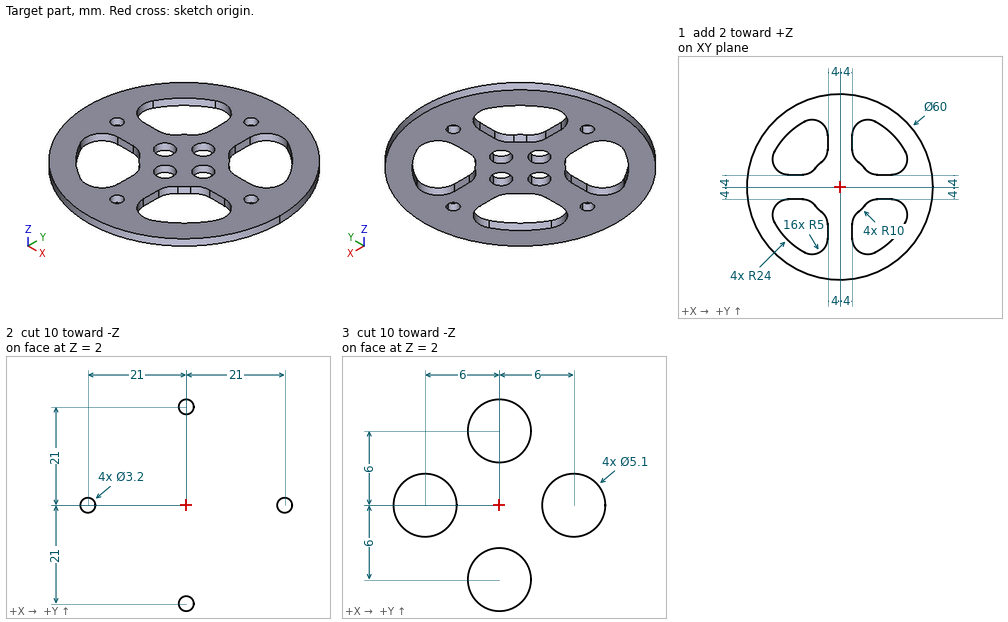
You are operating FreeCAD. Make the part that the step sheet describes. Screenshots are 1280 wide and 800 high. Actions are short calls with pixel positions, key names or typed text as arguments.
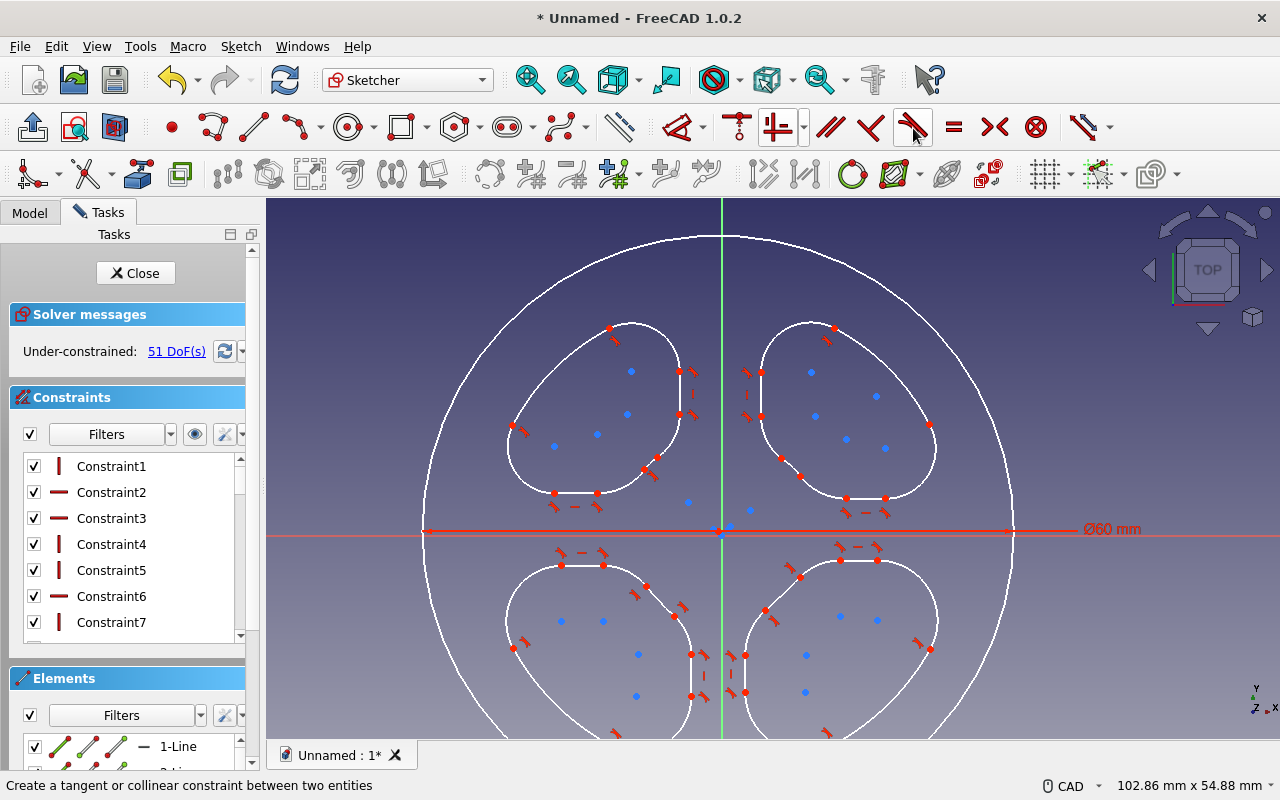
click(908, 390)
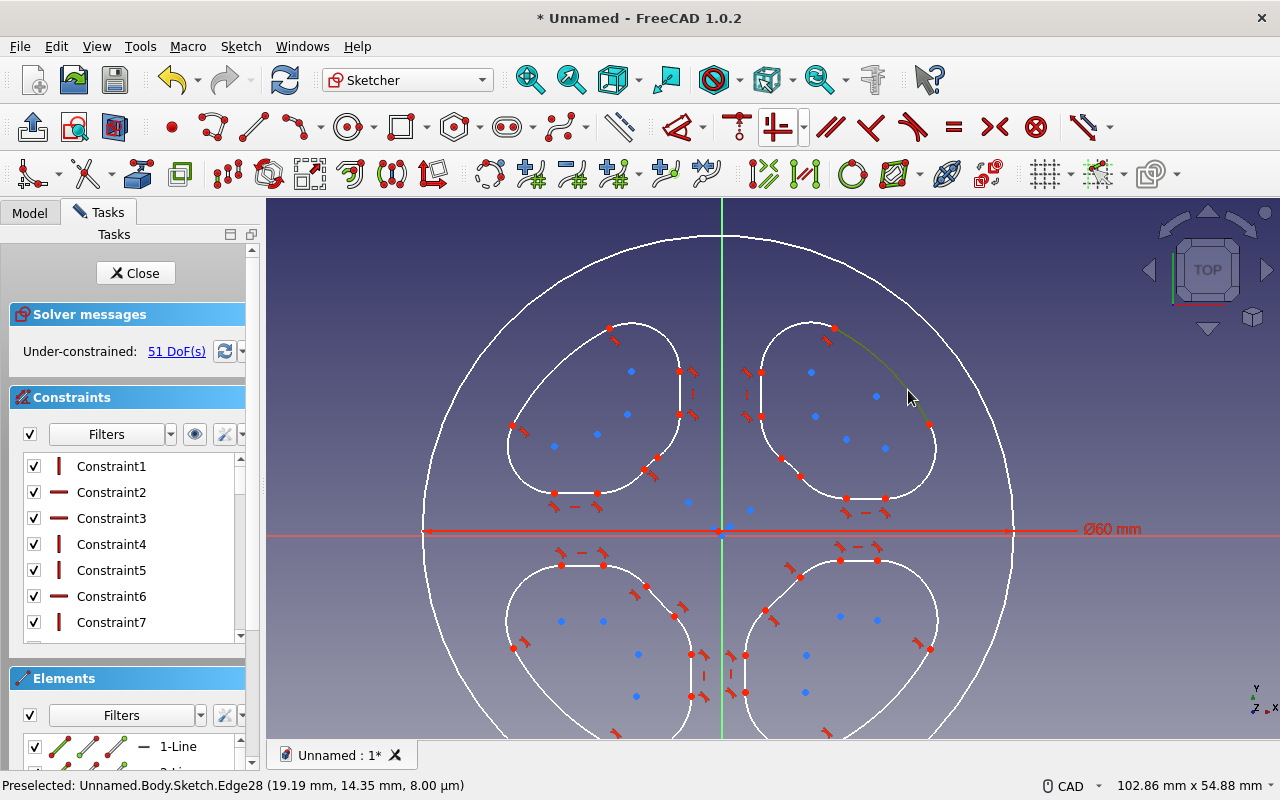
click(915, 489)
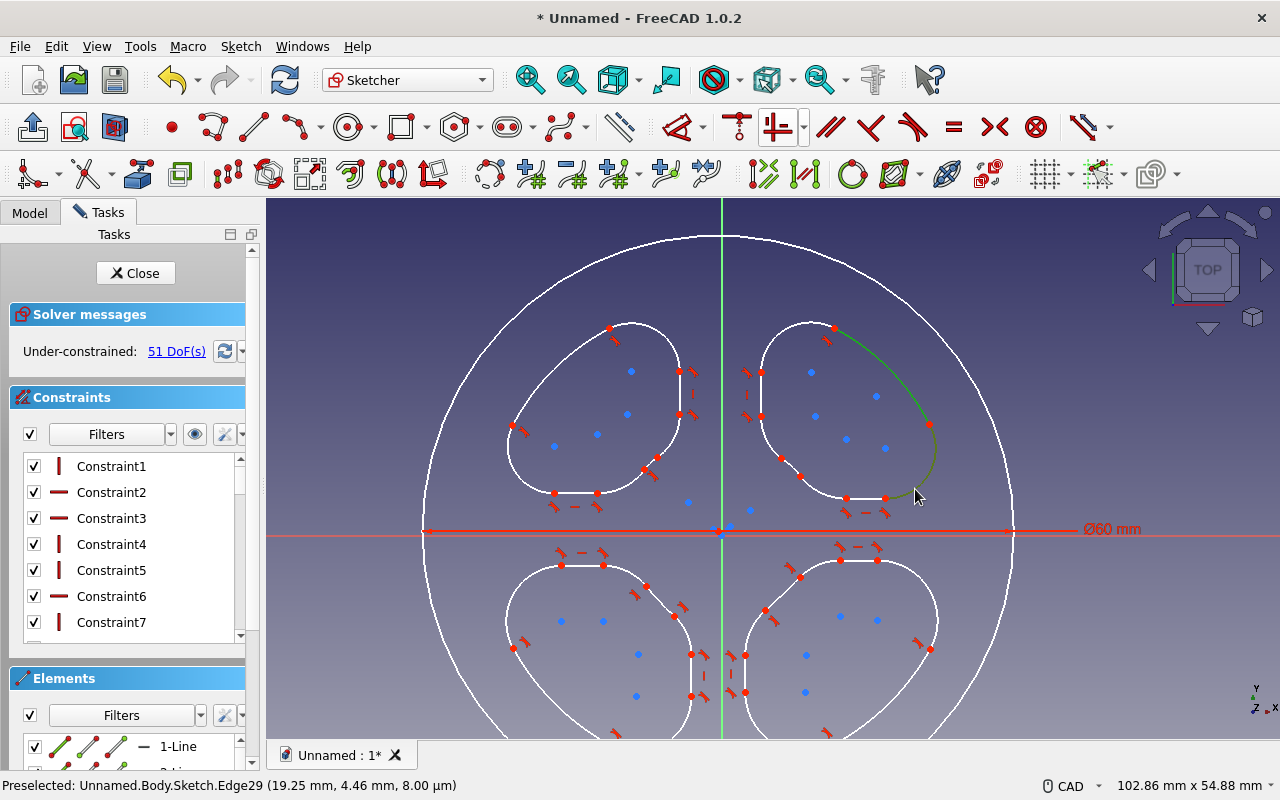
click(913, 128)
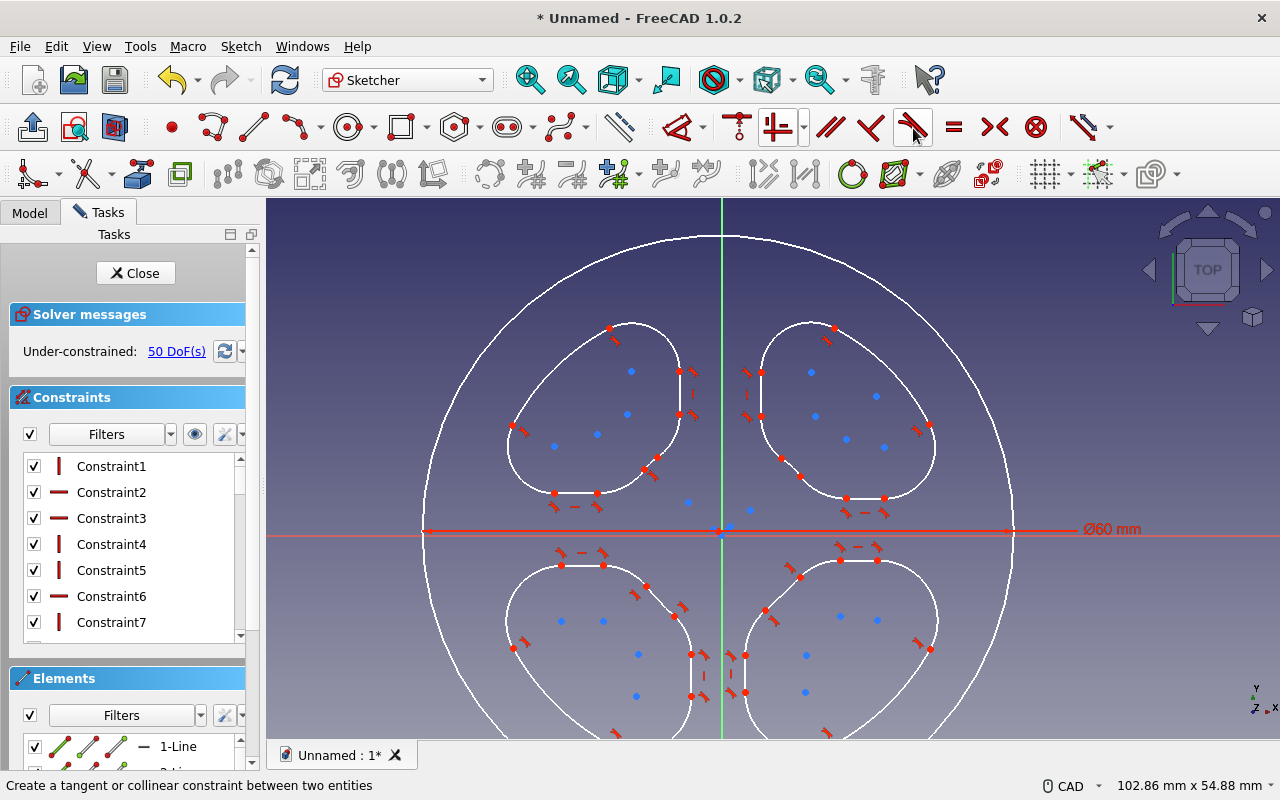
click(812, 488)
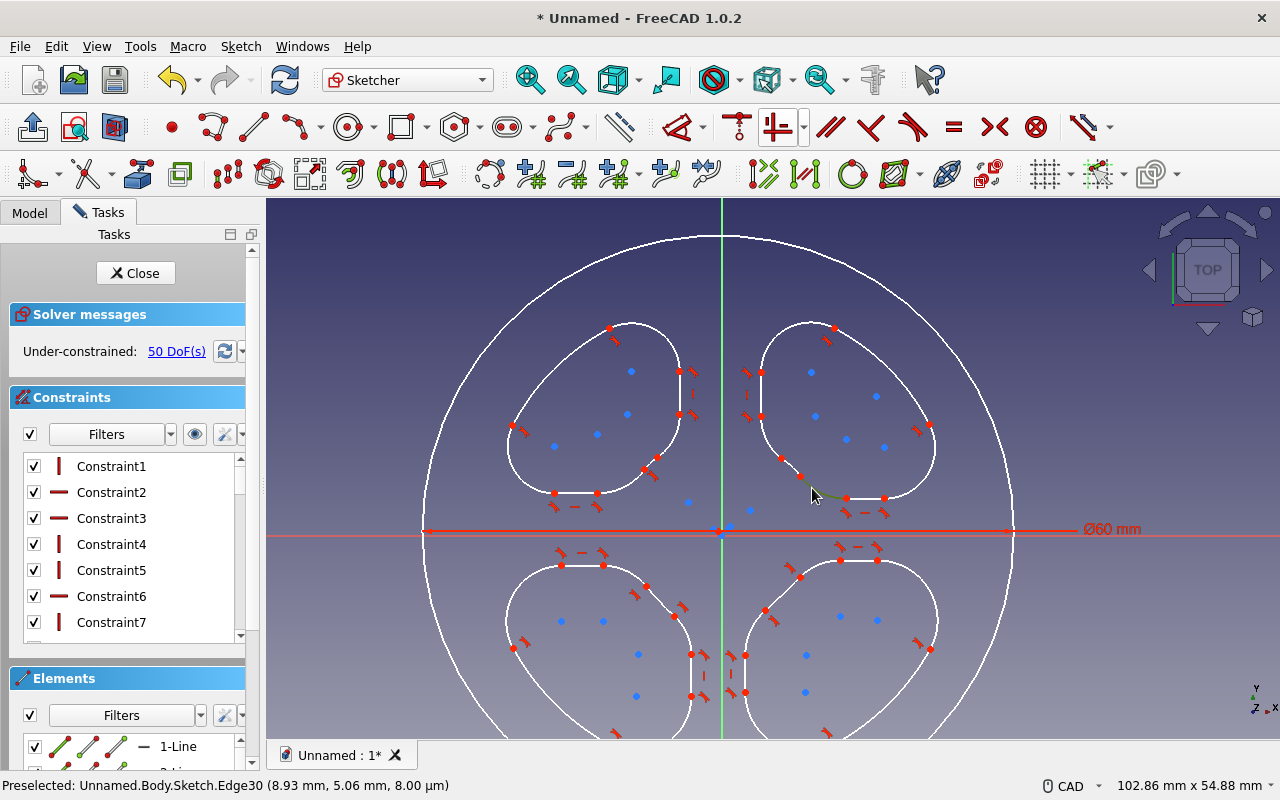
click(792, 467)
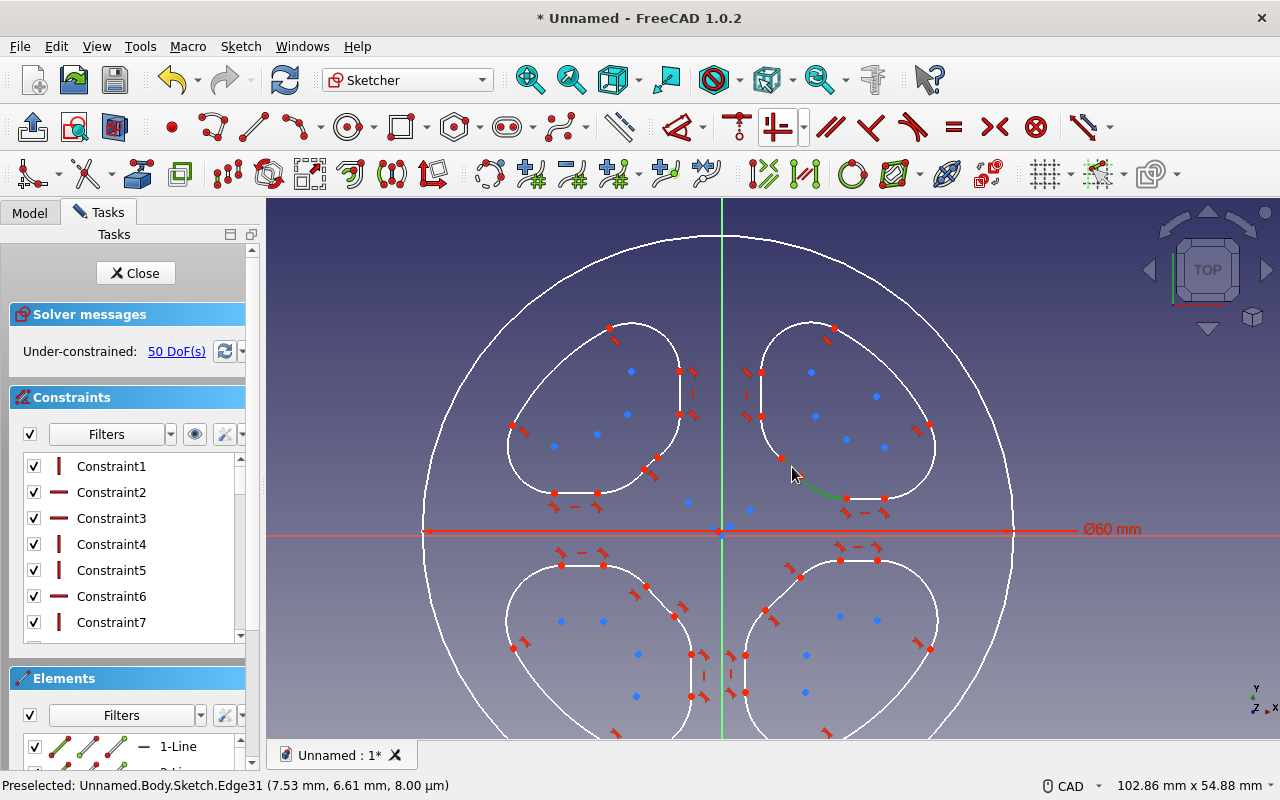
click(913, 128)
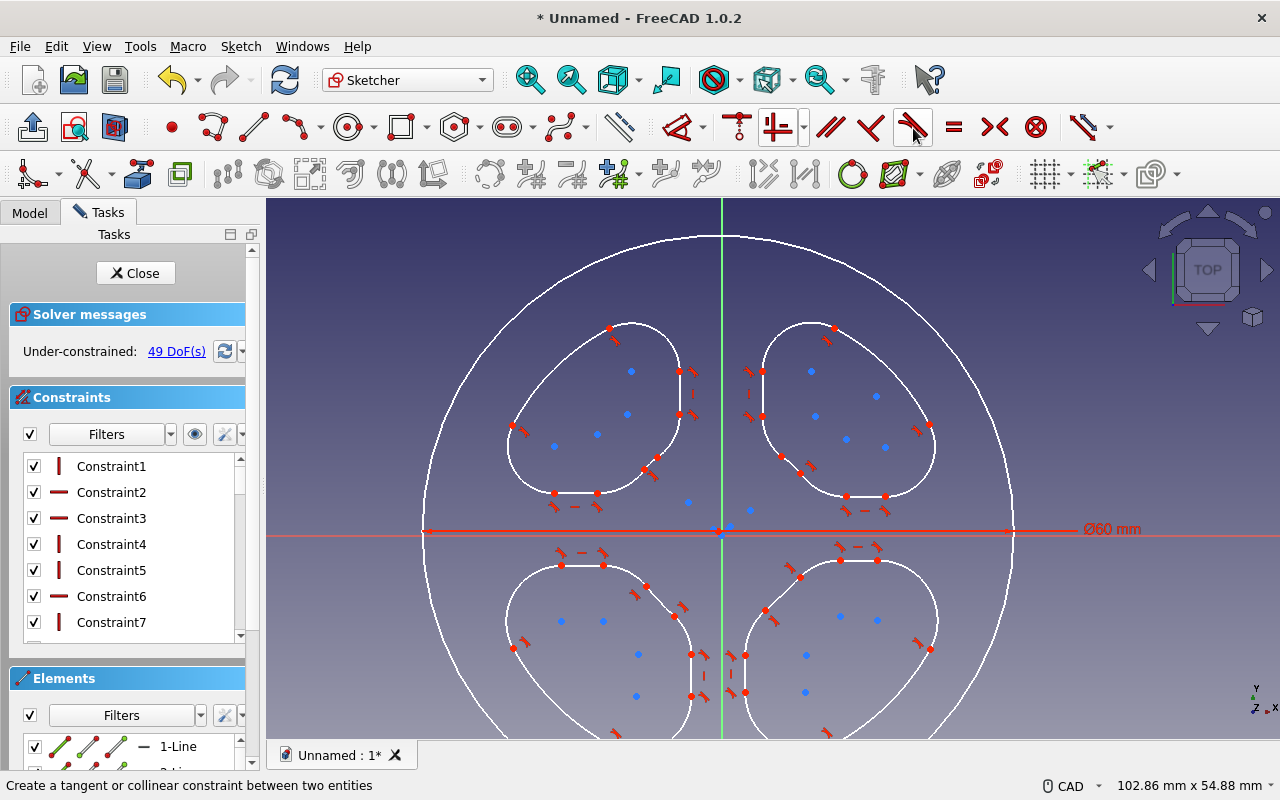
click(792, 464)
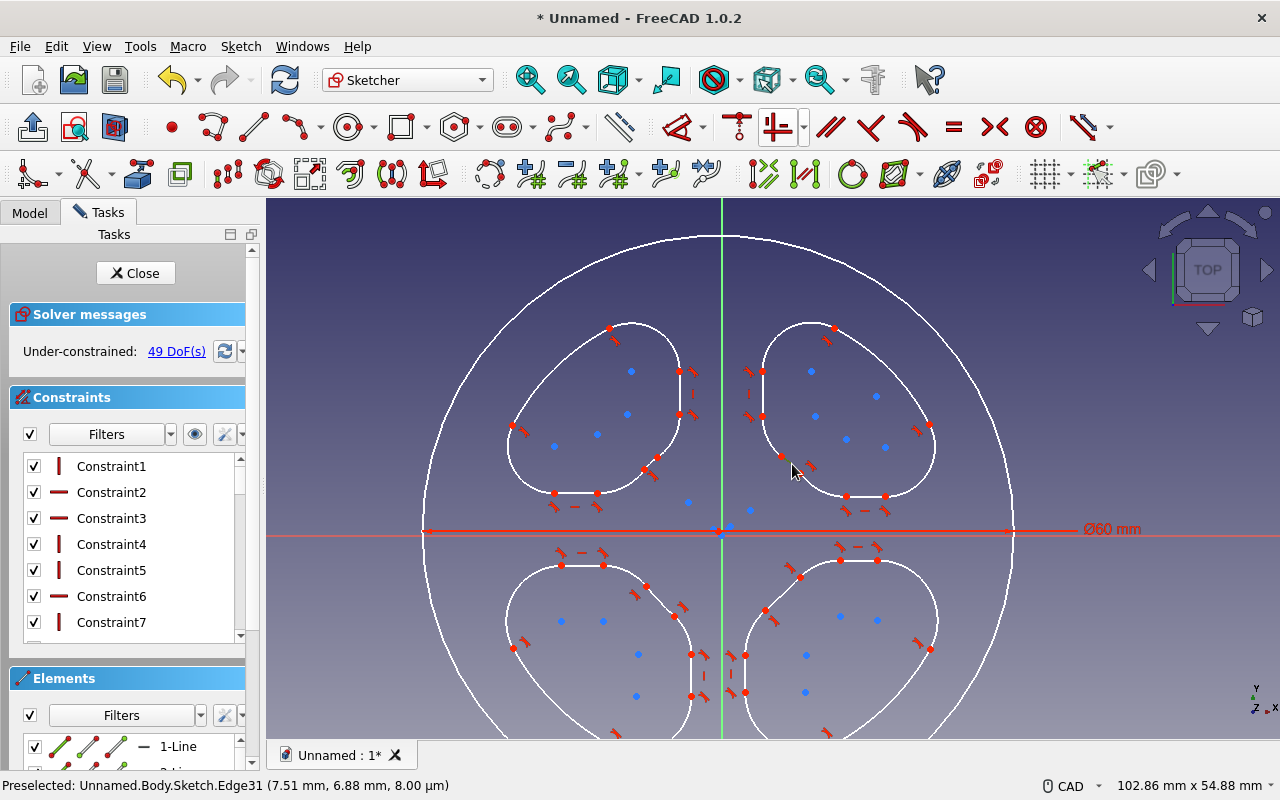
click(764, 430)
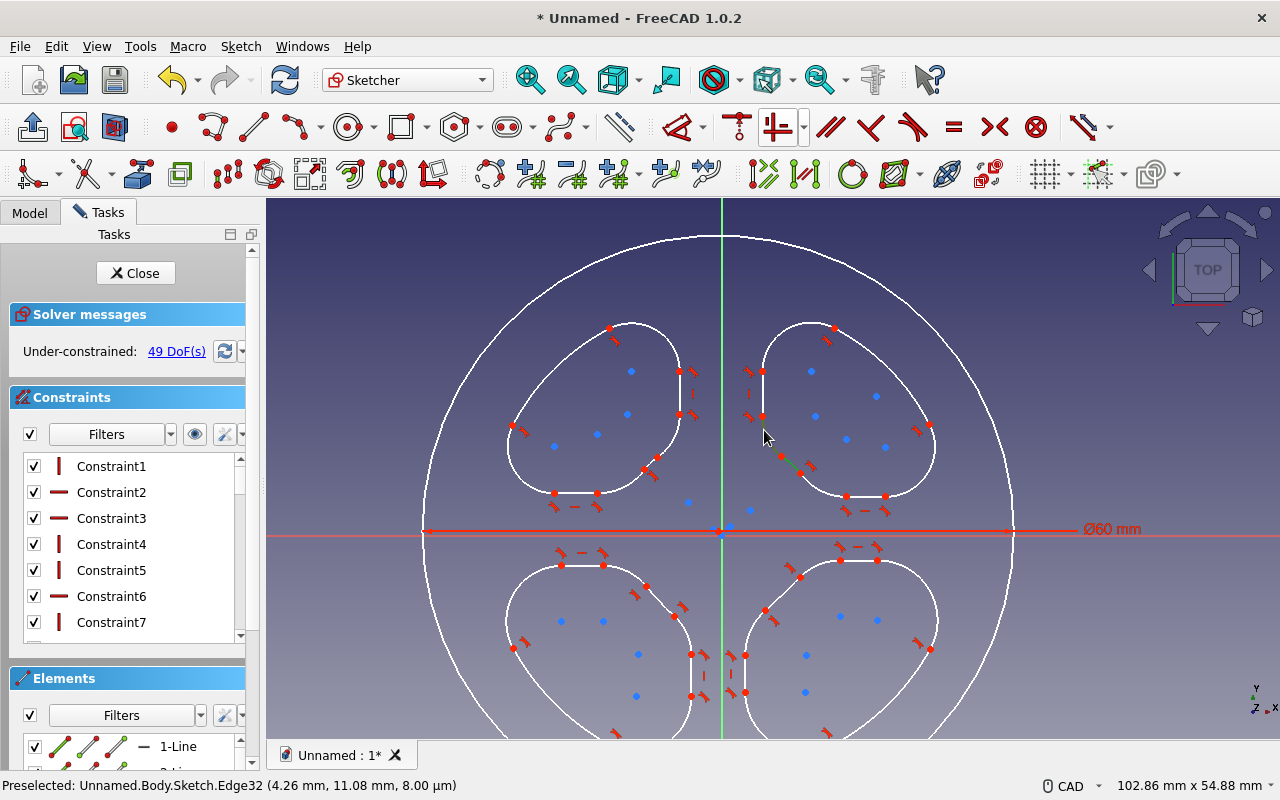
click(913, 128)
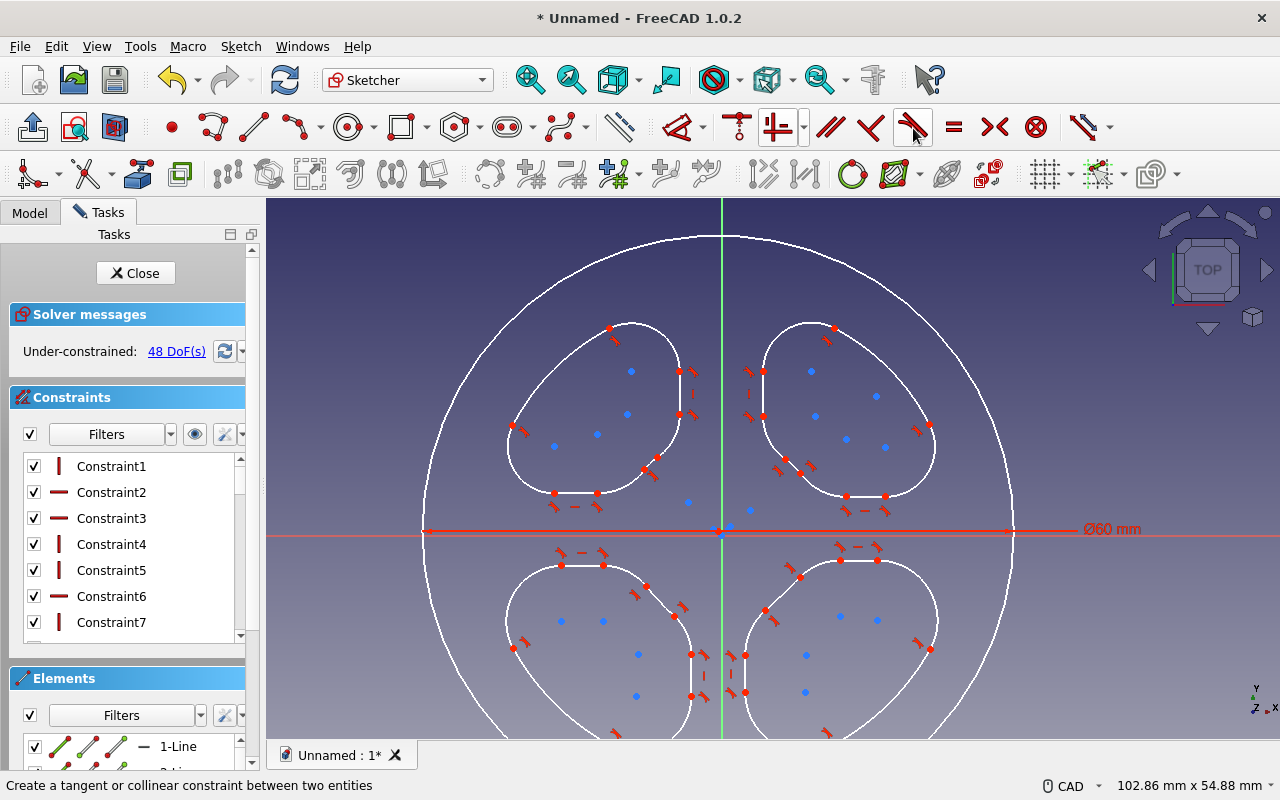
click(927, 322)